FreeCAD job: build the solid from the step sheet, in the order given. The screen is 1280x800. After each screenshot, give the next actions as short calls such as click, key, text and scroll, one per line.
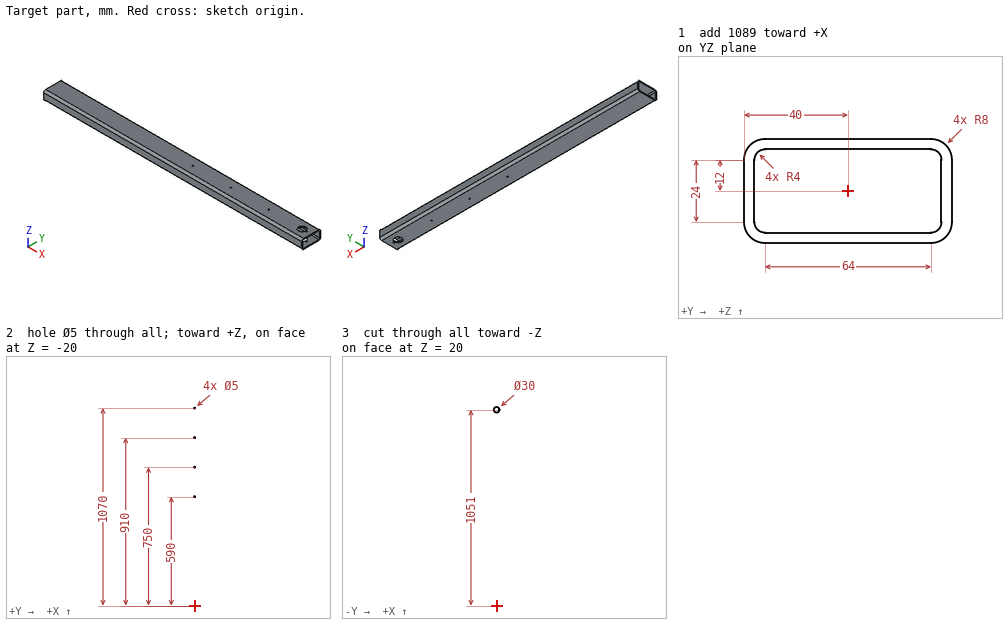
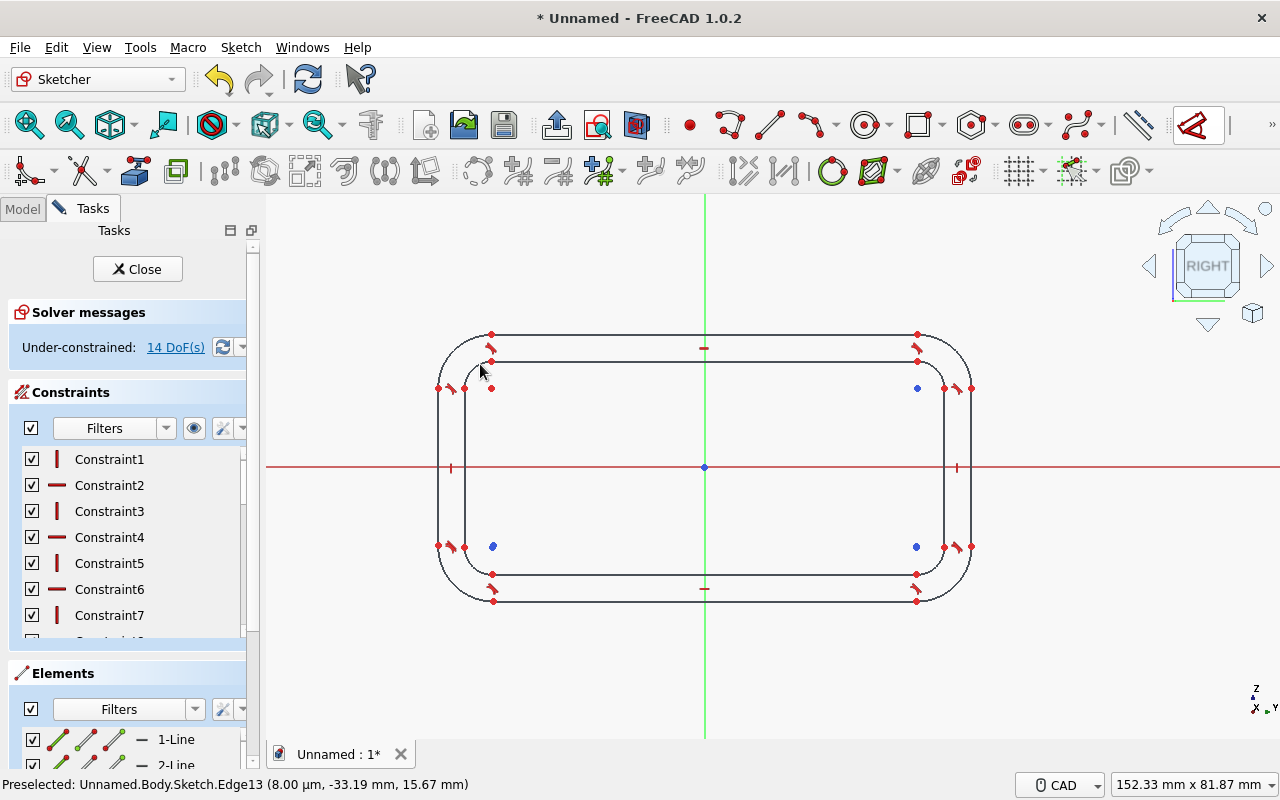
click(966, 364)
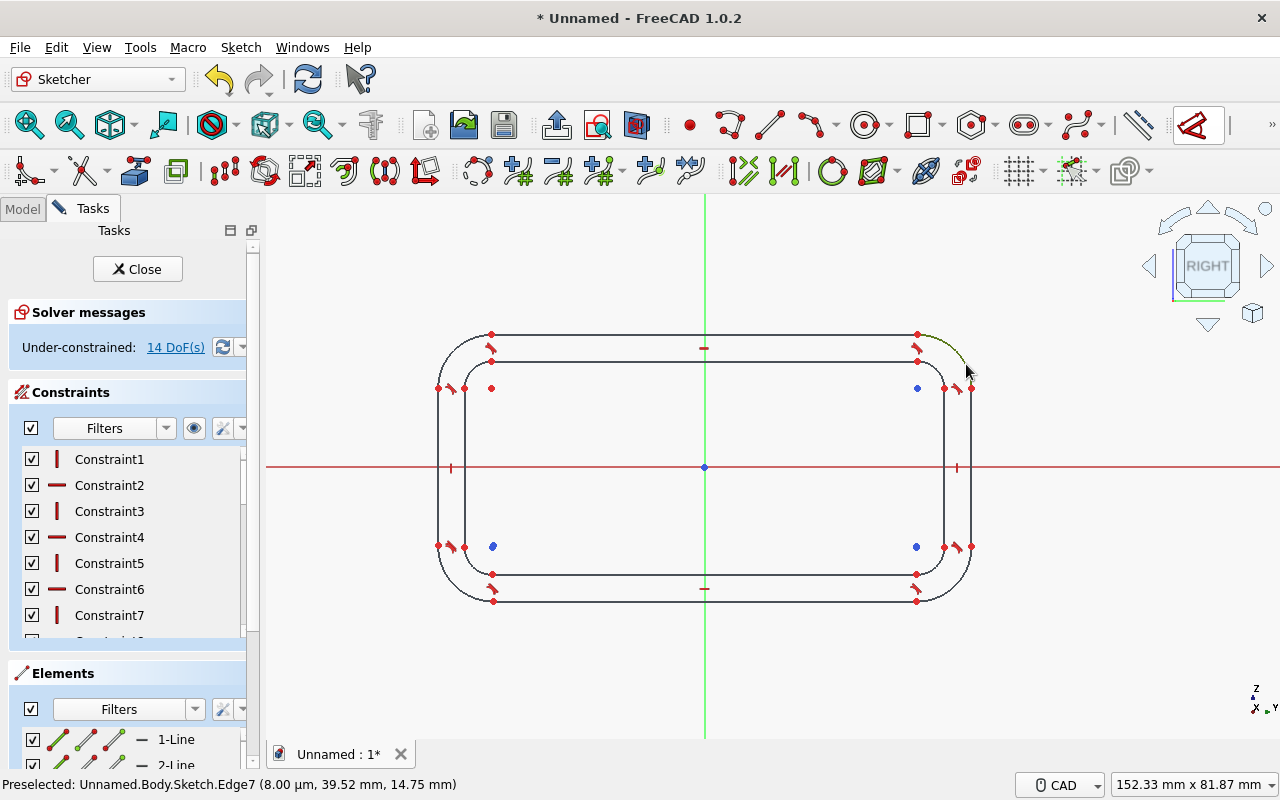
click(941, 376)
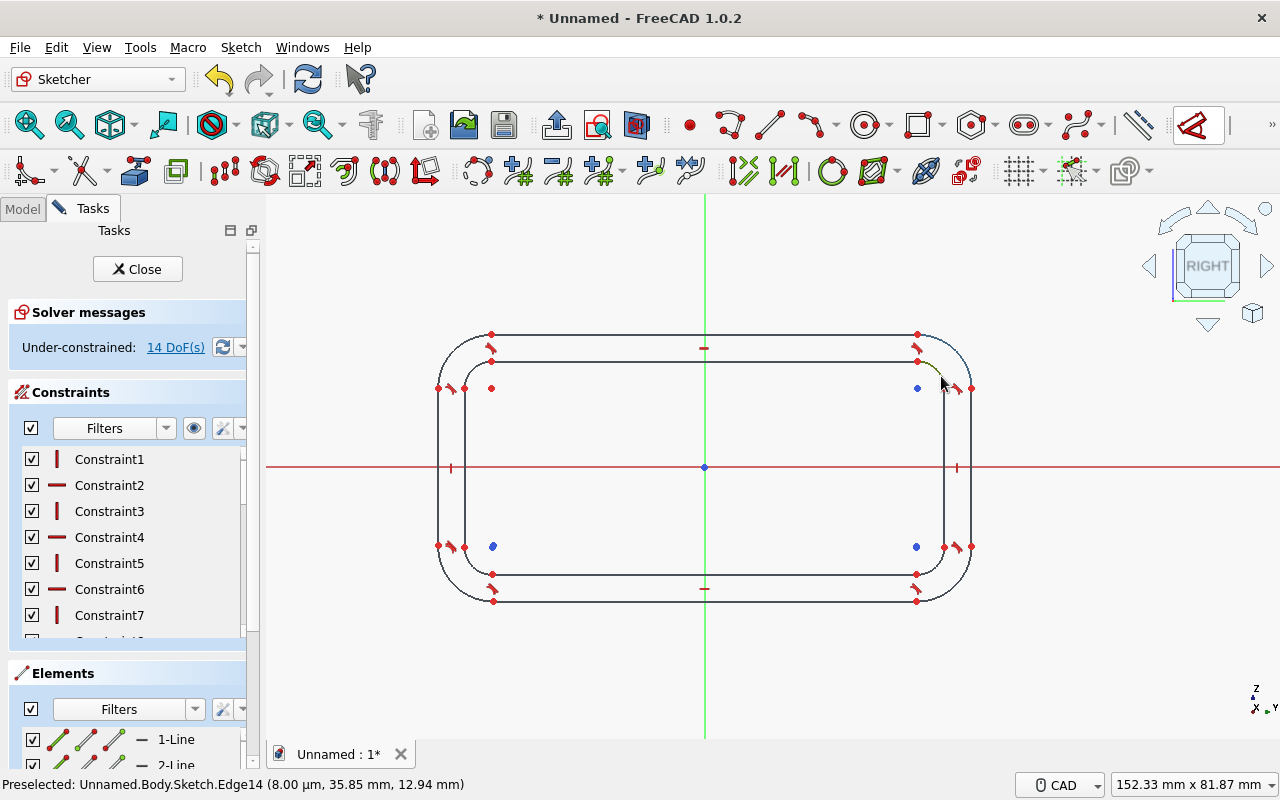
key(c)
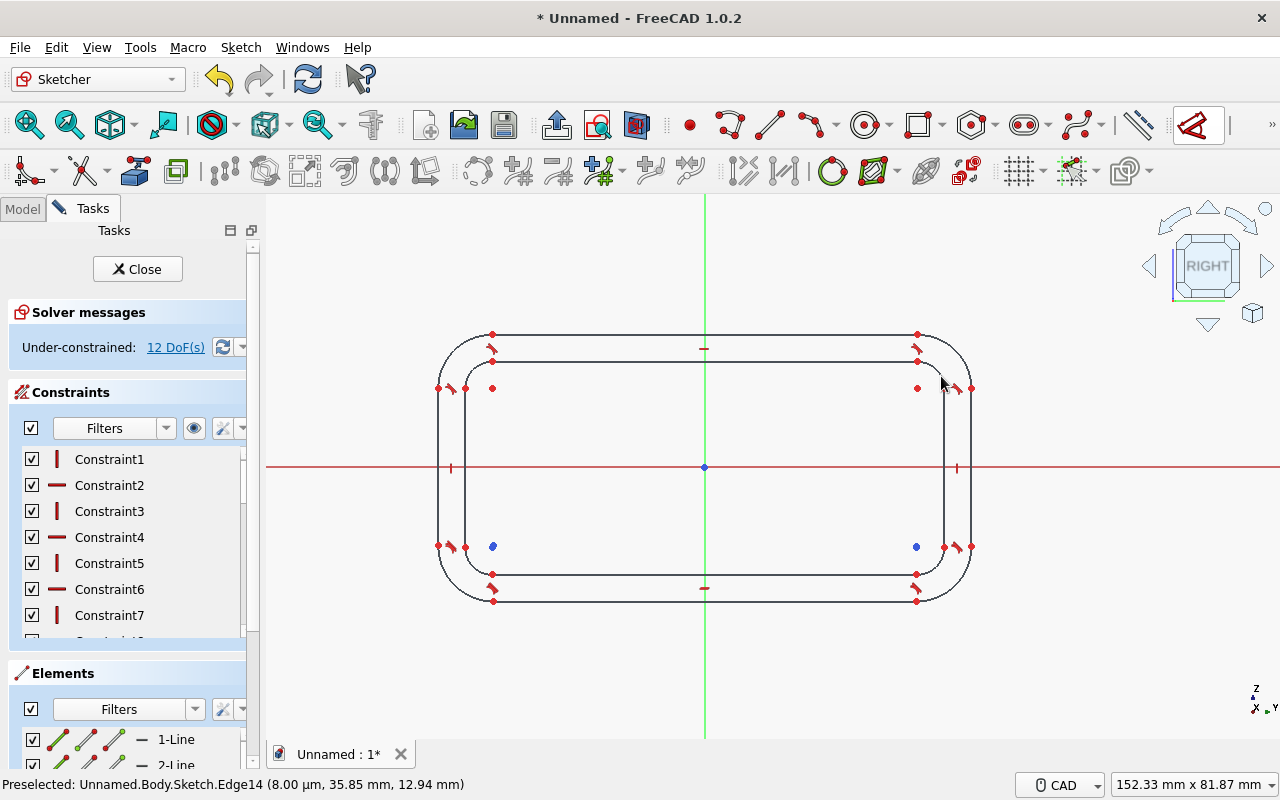
click(941, 596)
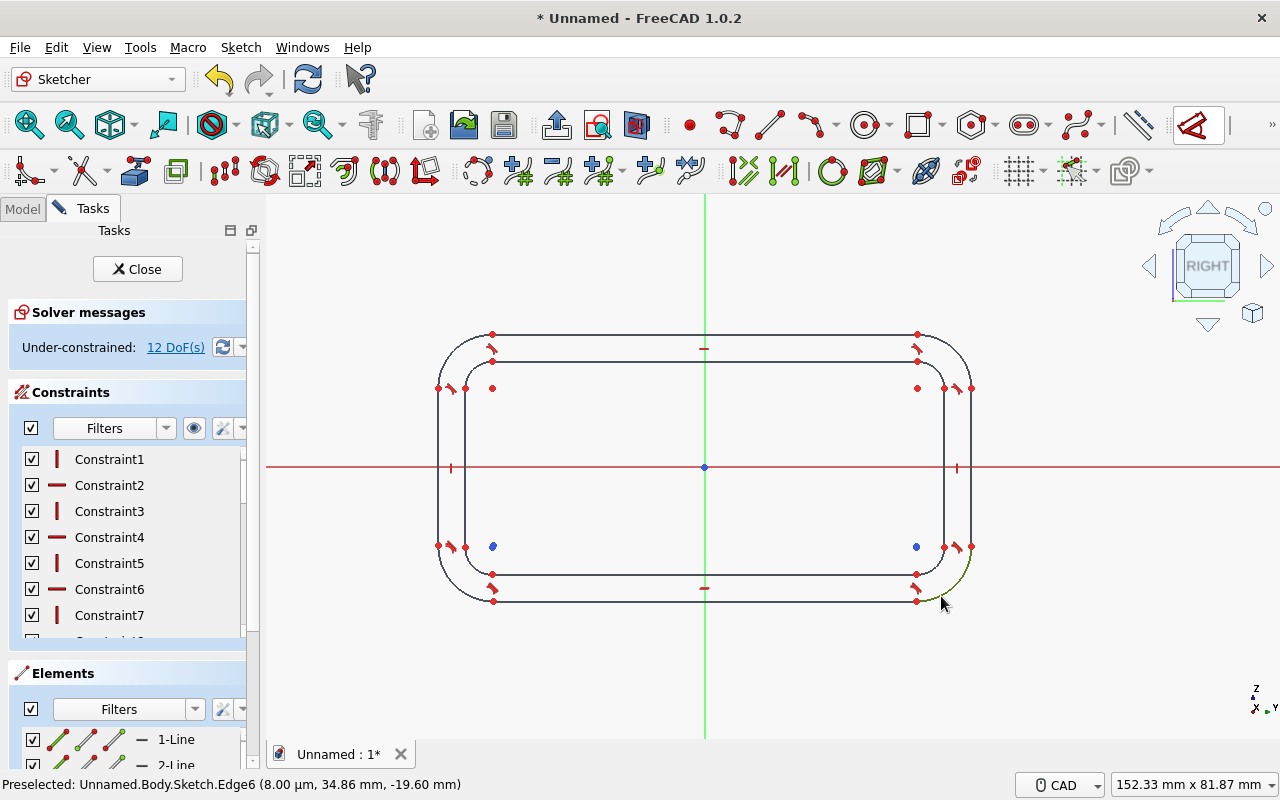
click(929, 572)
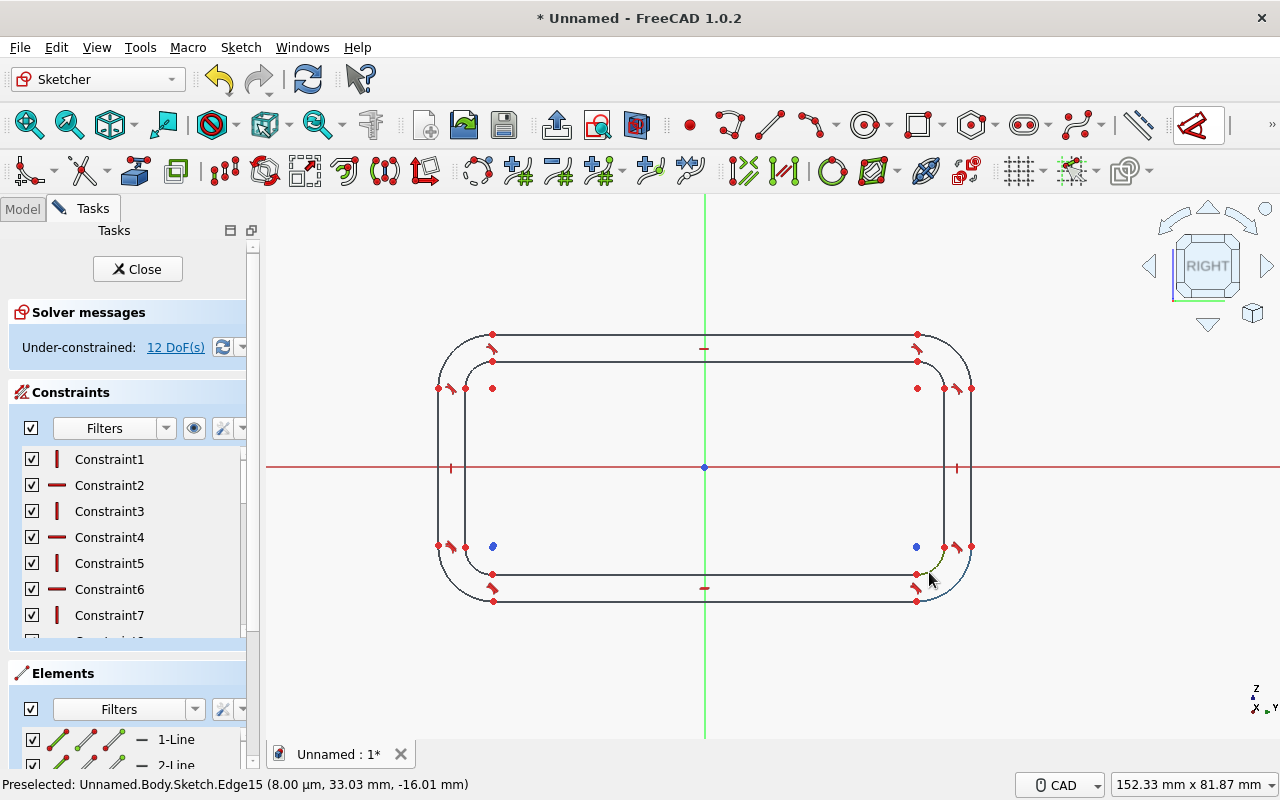
key(c)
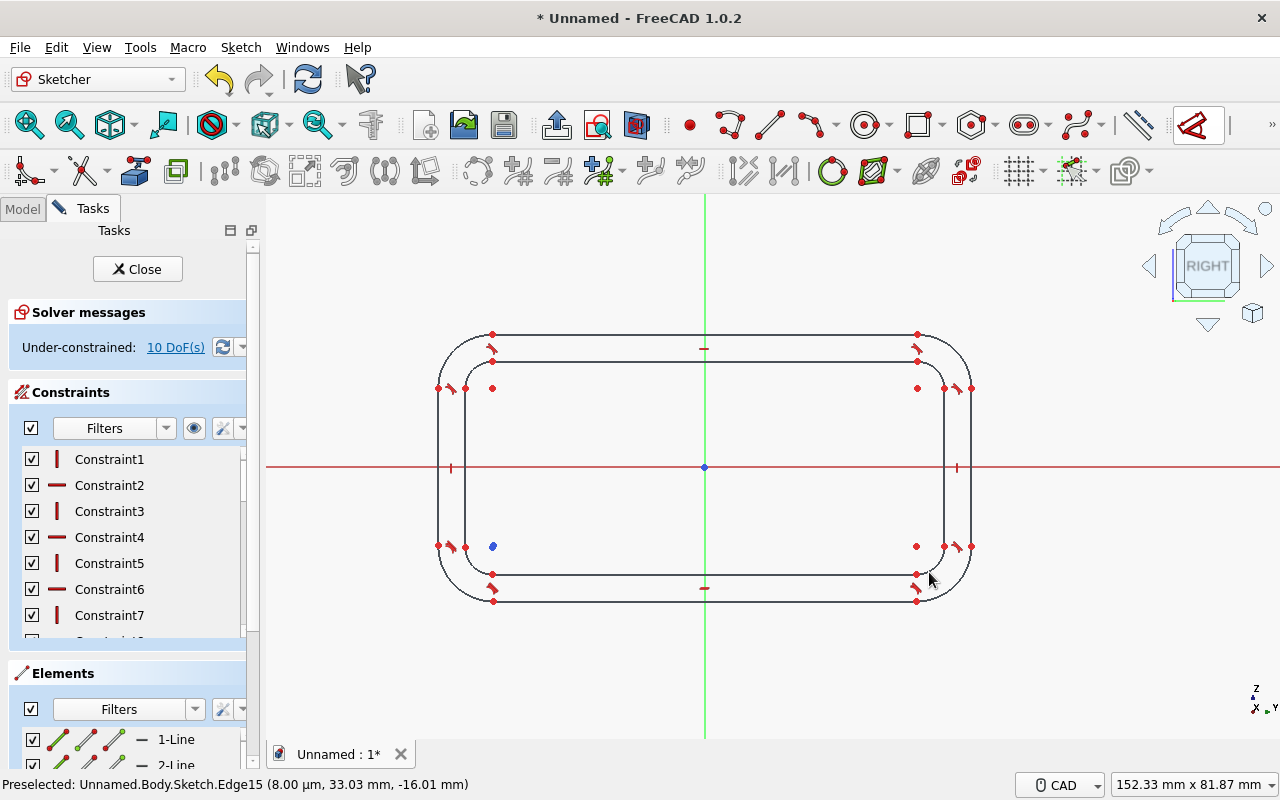
click(444, 571)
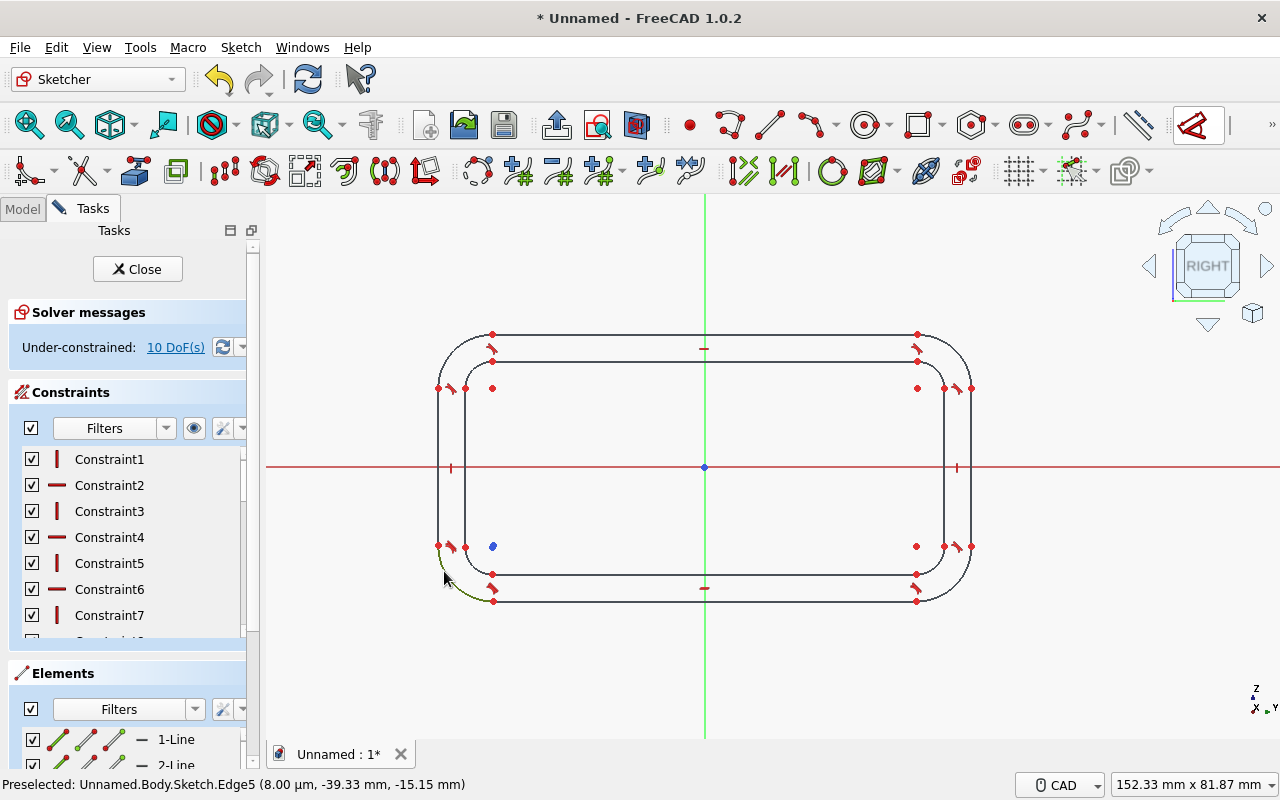
click(941, 596)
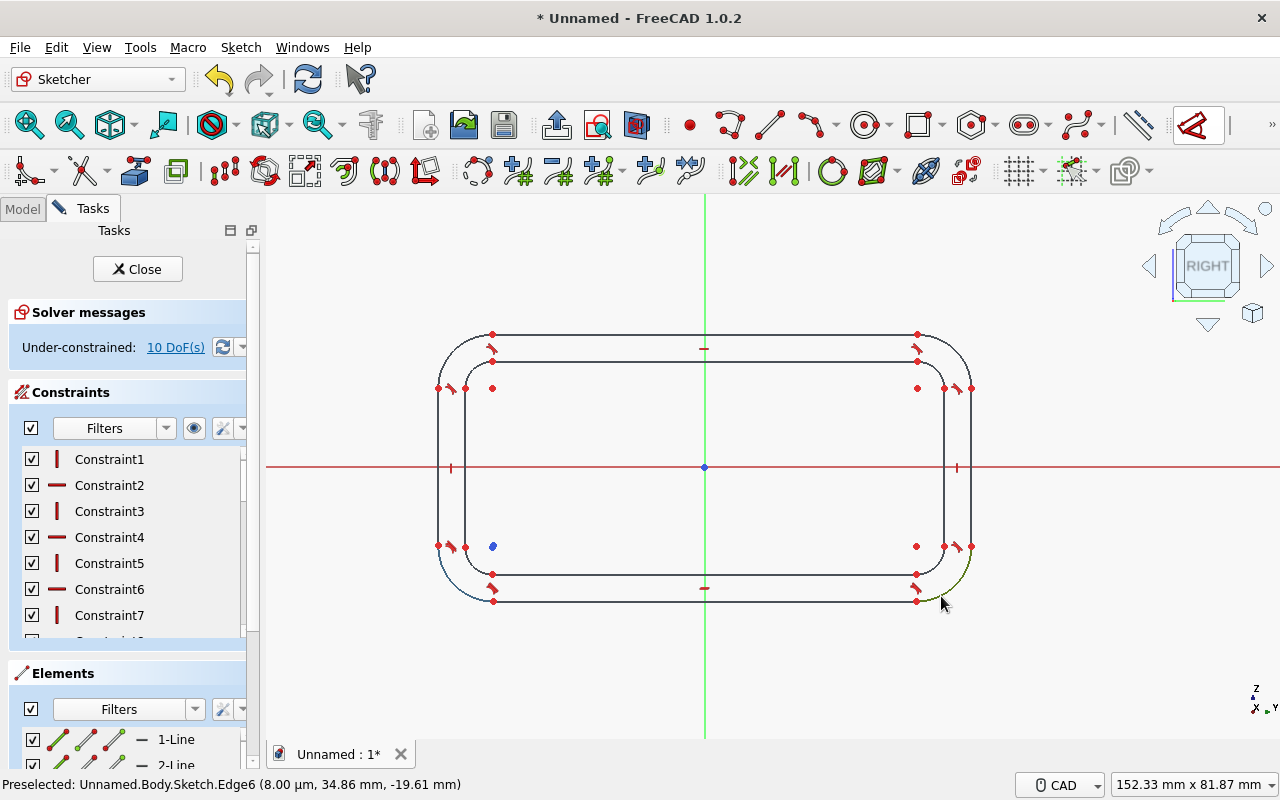
click(965, 364)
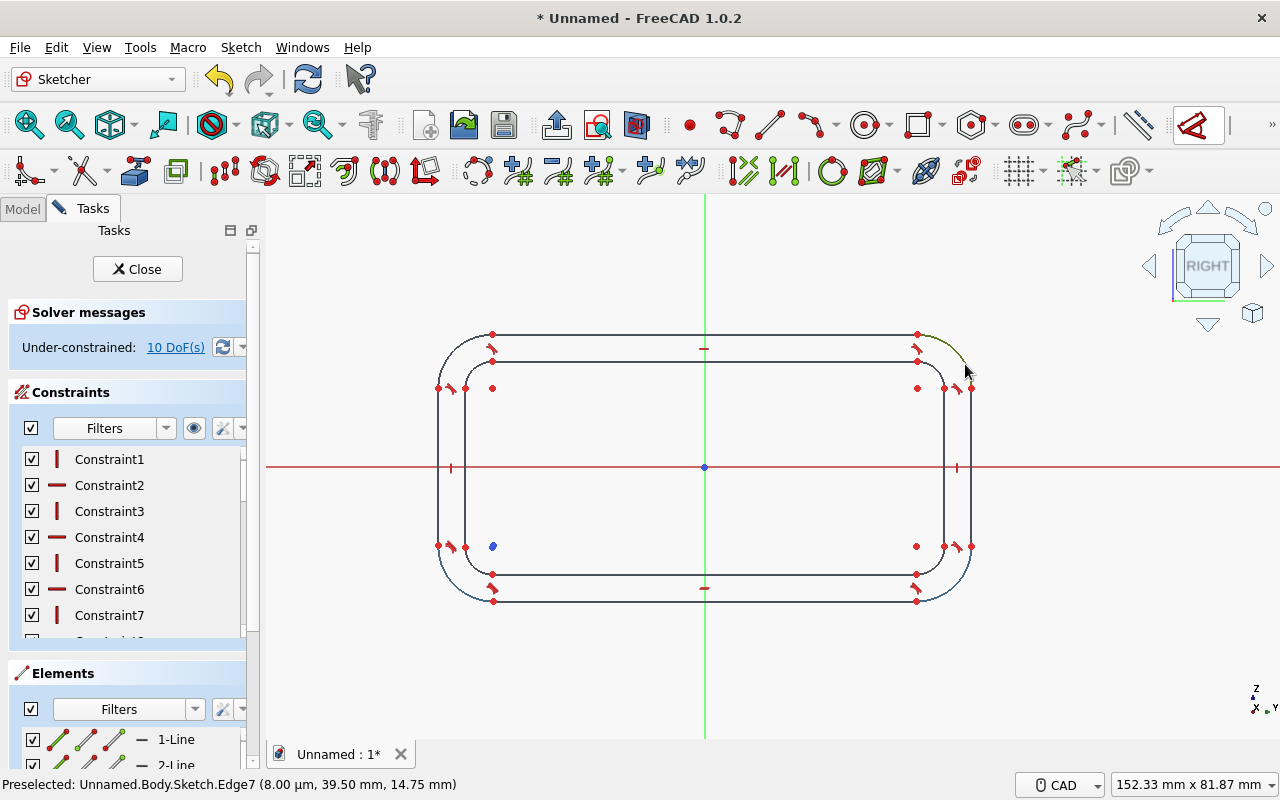
click(468, 341)